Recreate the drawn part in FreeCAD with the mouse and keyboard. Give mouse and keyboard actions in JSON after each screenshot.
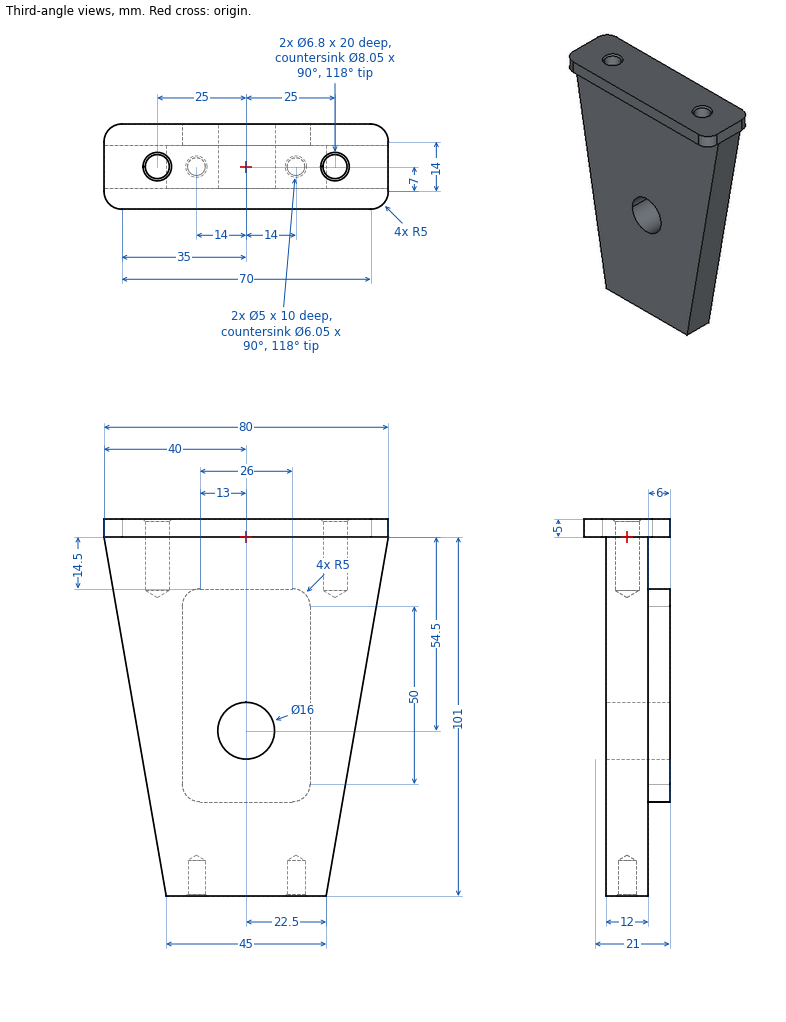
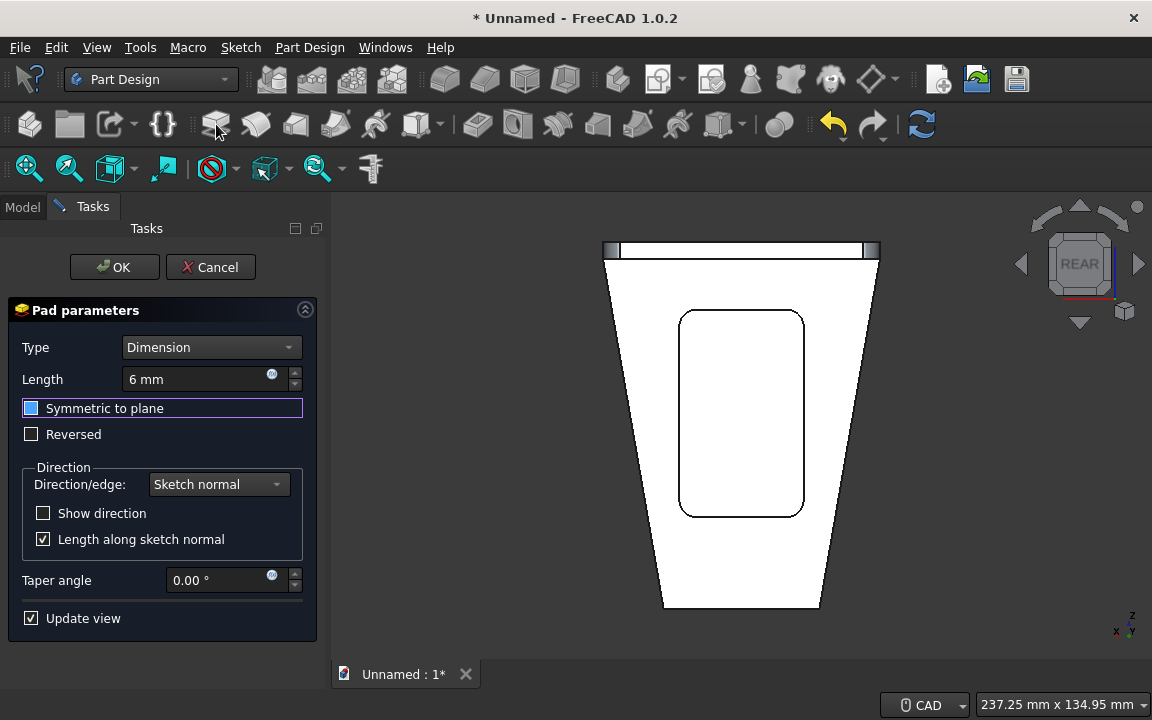
{"action": "left_click", "coordinate": [115, 267]}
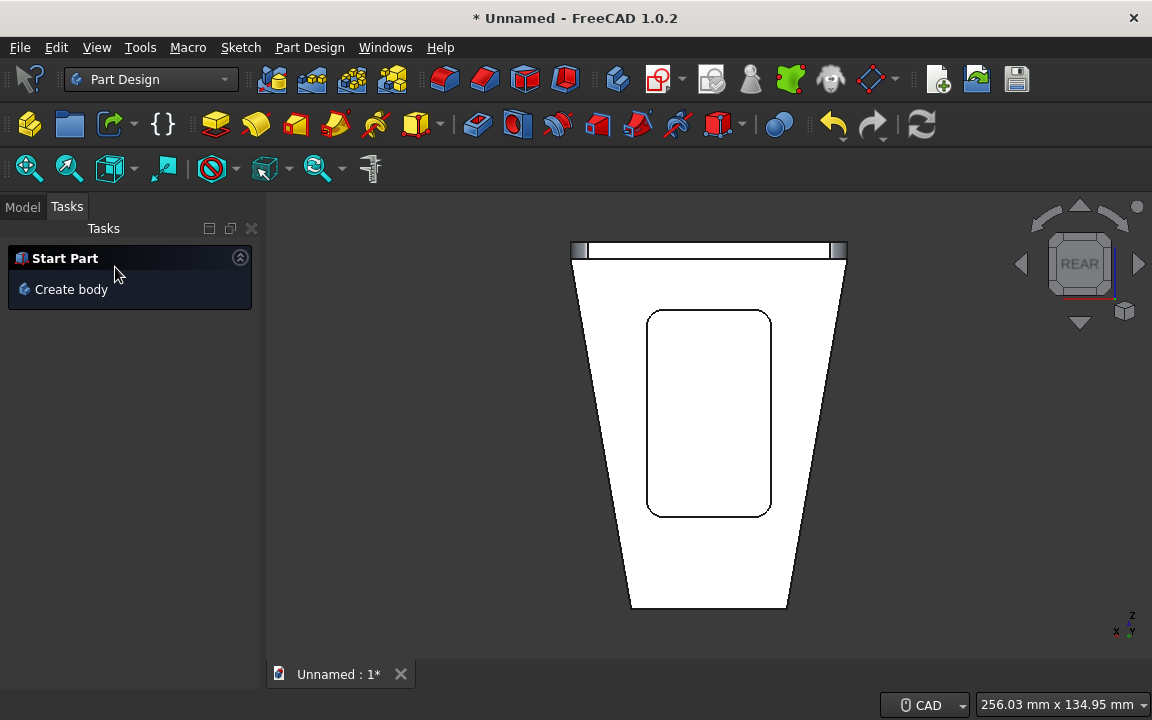
{"action": "left_click", "coordinate": [709, 383]}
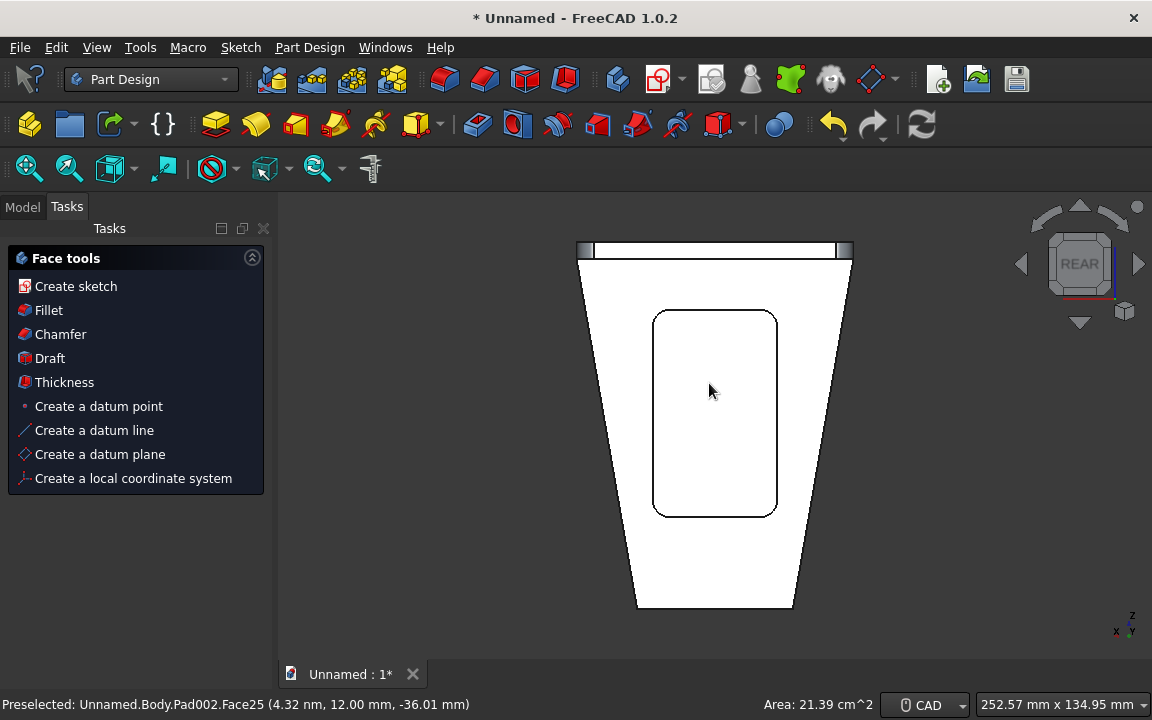
{"action": "left_click", "coordinate": [658, 80]}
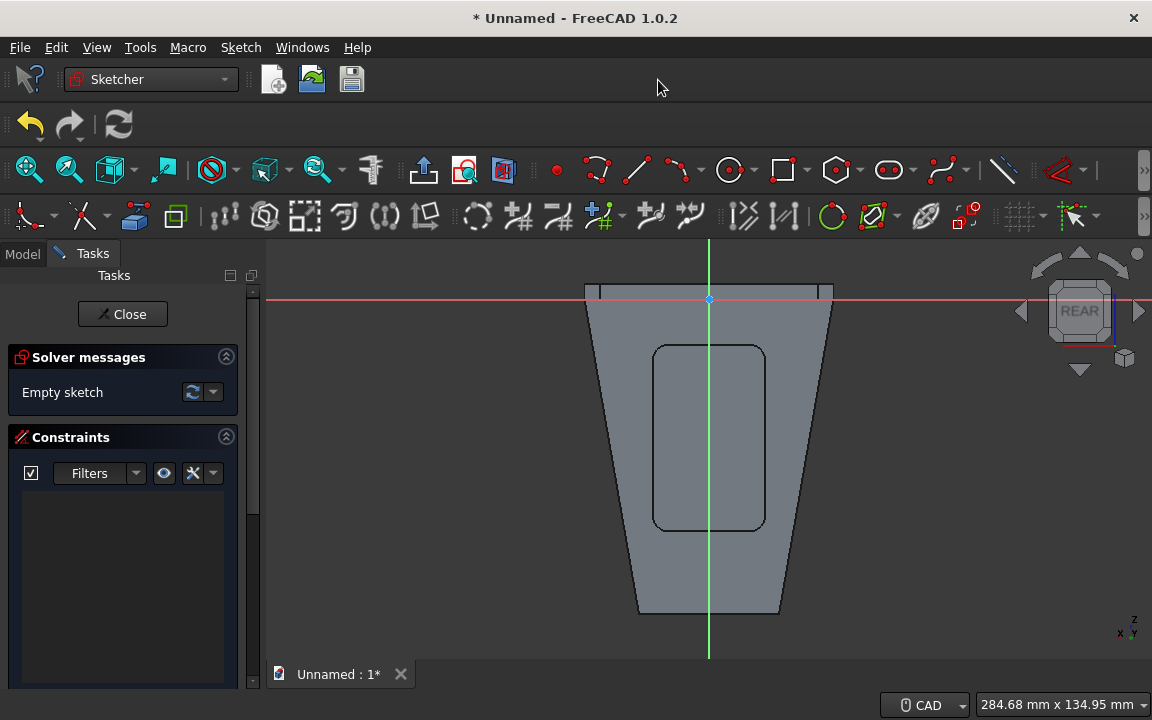
{"action": "scroll", "coordinate": [726, 474], "scroll_direction": "up", "scroll_amount": 8}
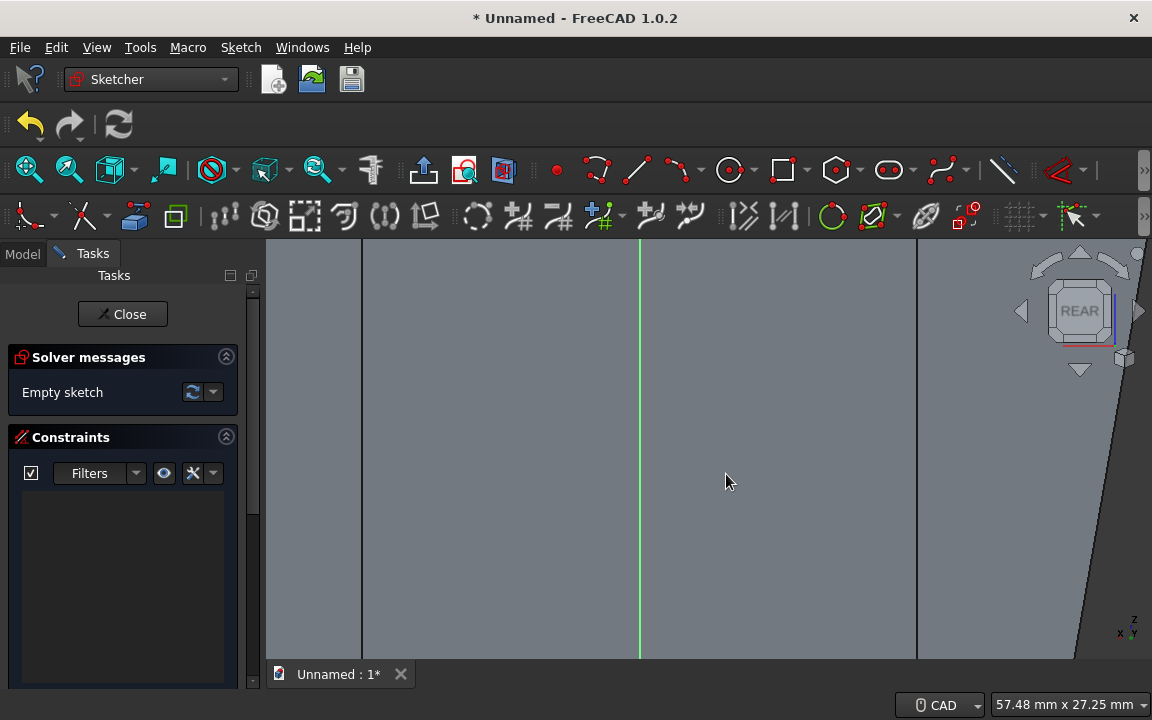
{"action": "left_click", "coordinate": [730, 170]}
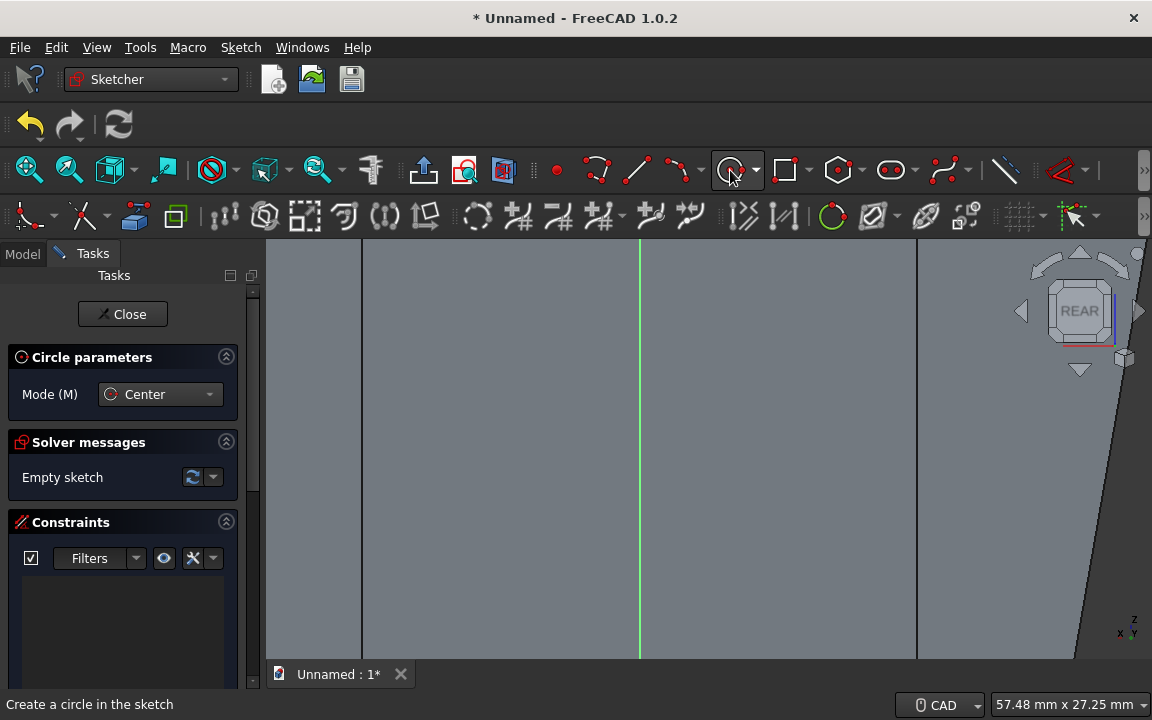
{"action": "left_click", "coordinate": [640, 448]}
{"action": "mouse_move", "coordinate": [727, 361]}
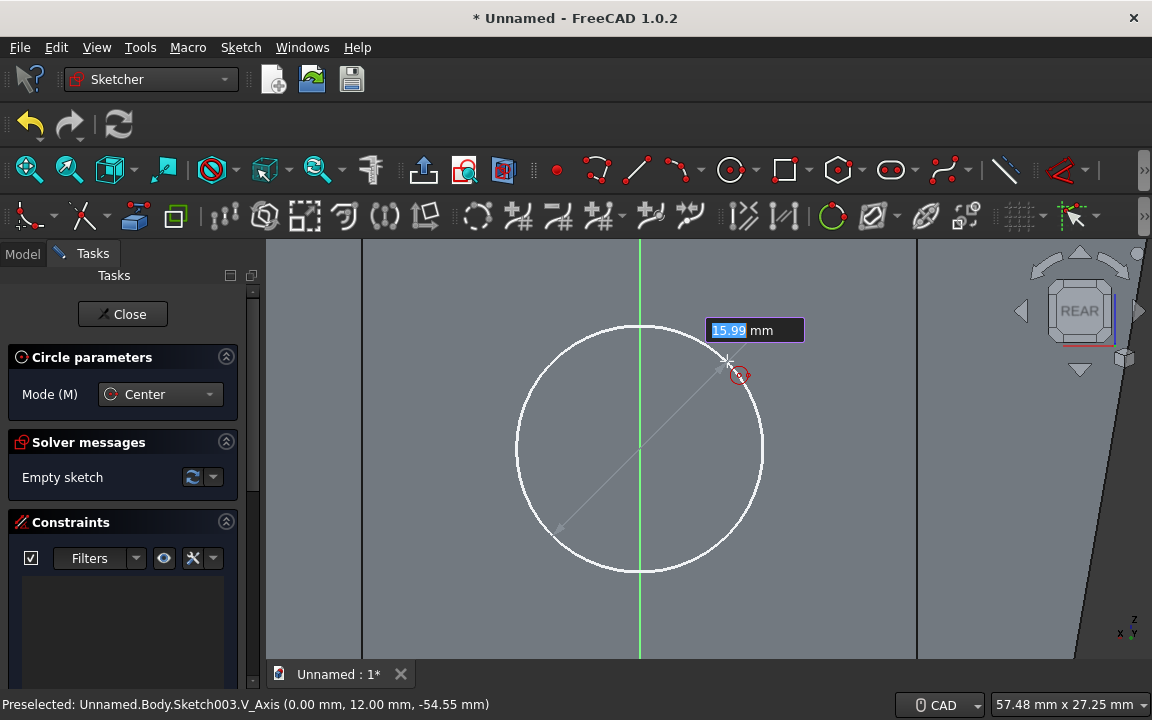
{"action": "type", "text": "16"}
{"action": "key", "text": "Return"}
{"action": "key", "text": "Escape"}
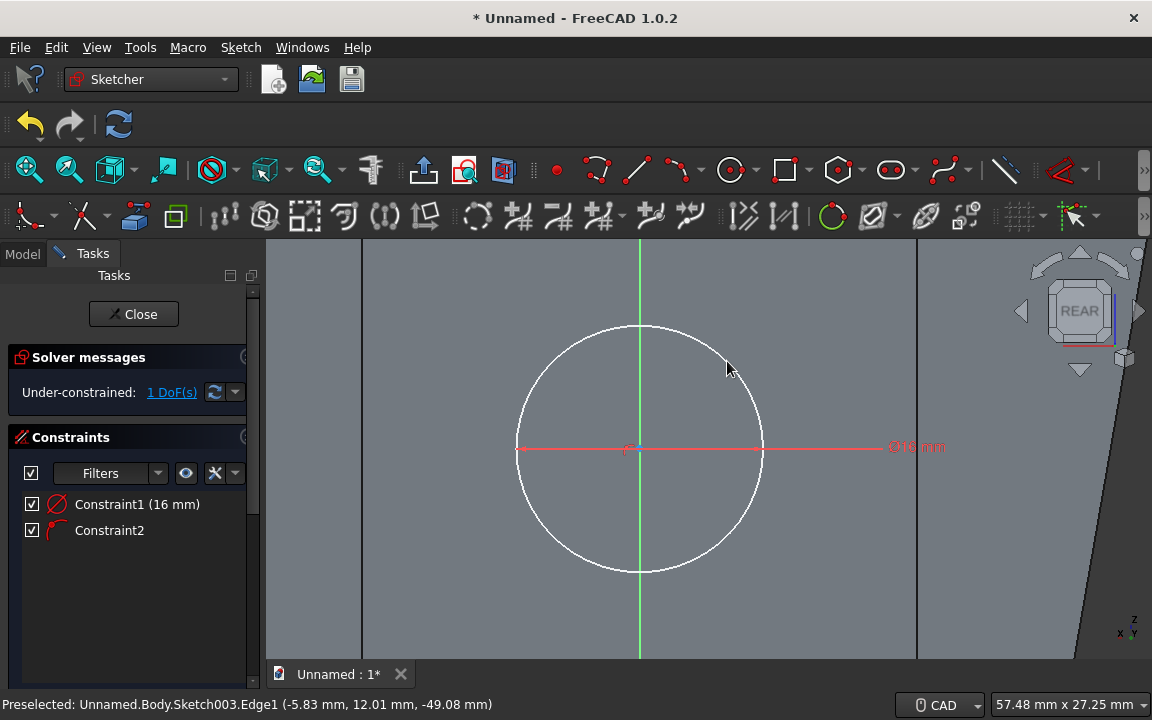
{"action": "left_click", "coordinate": [1060, 170]}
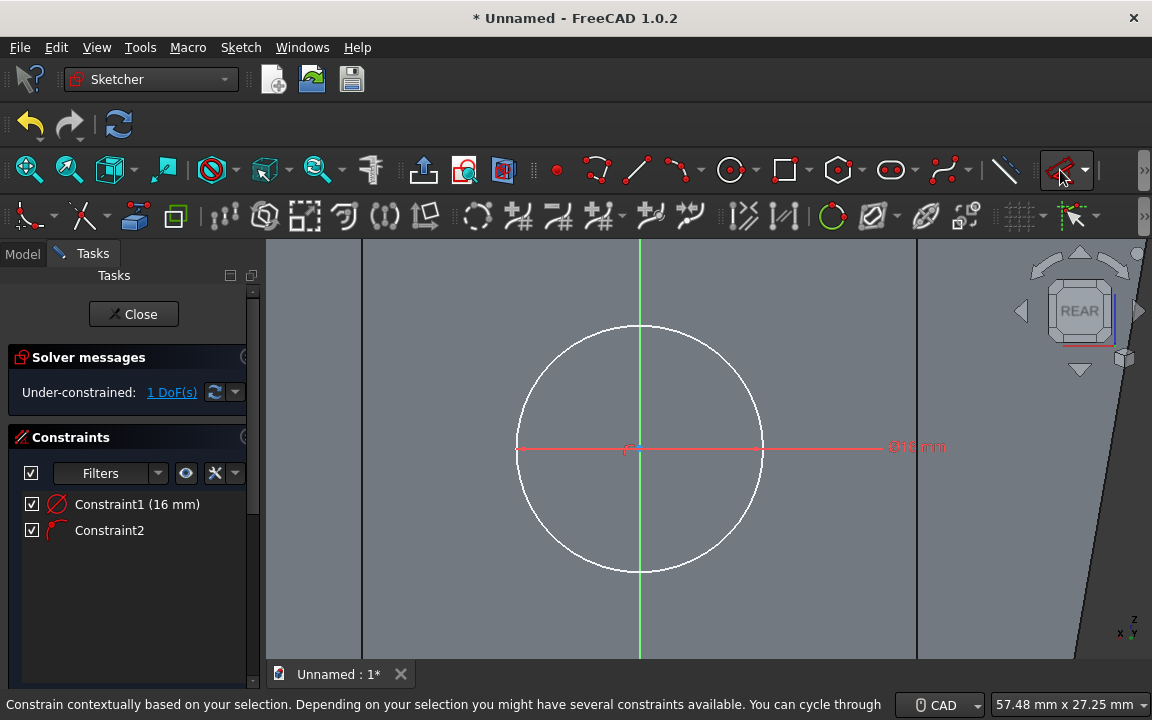
{"action": "left_click", "coordinate": [640, 449]}
{"action": "left_click", "coordinate": [674, 358]}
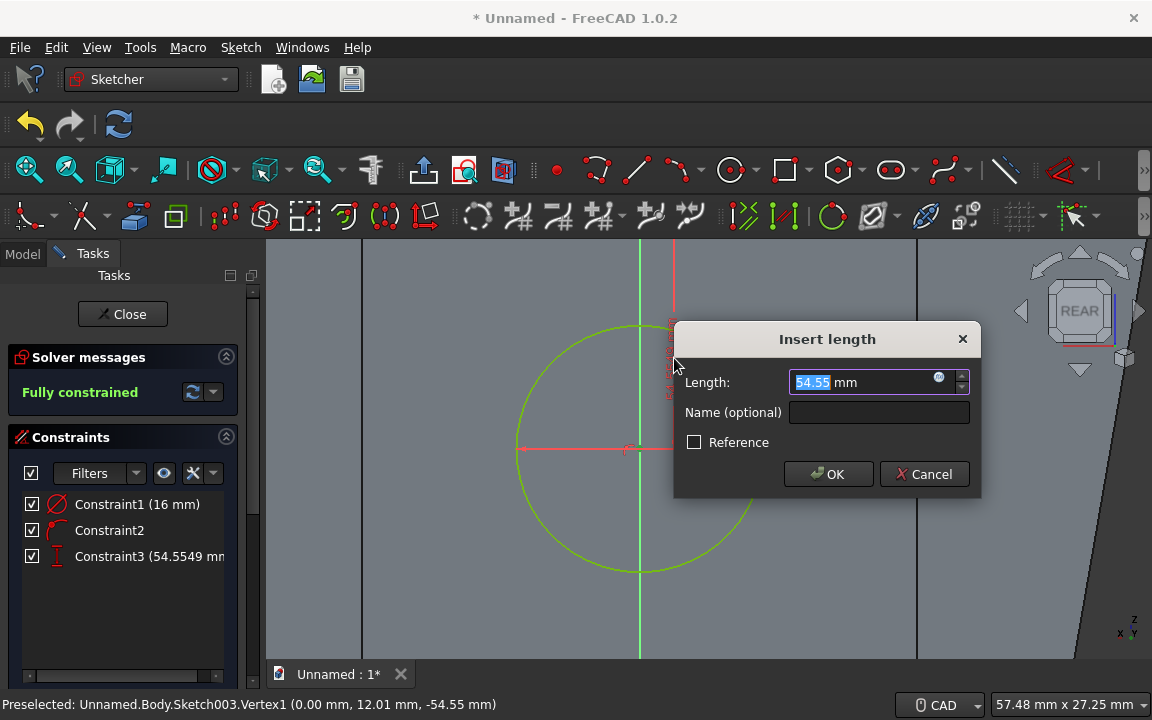
{"action": "type", "text": "54.5"}
{"action": "key", "text": "Return"}
{"action": "key", "text": "Escape"}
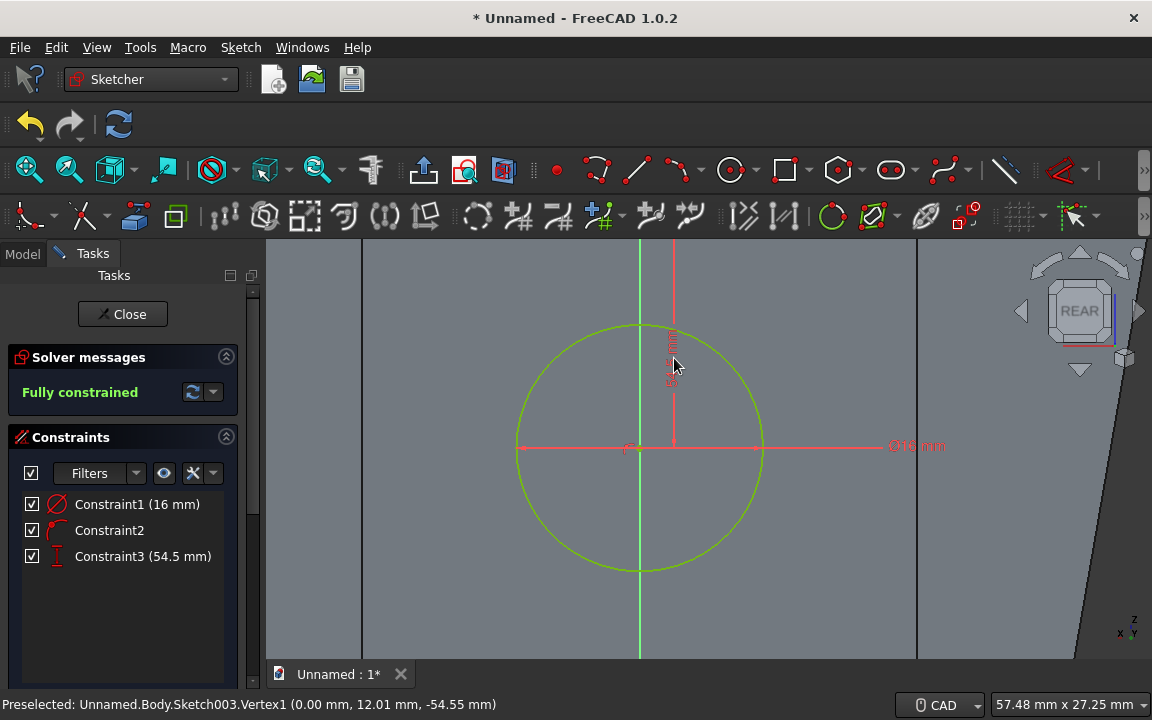
{"action": "left_click", "coordinate": [123, 314]}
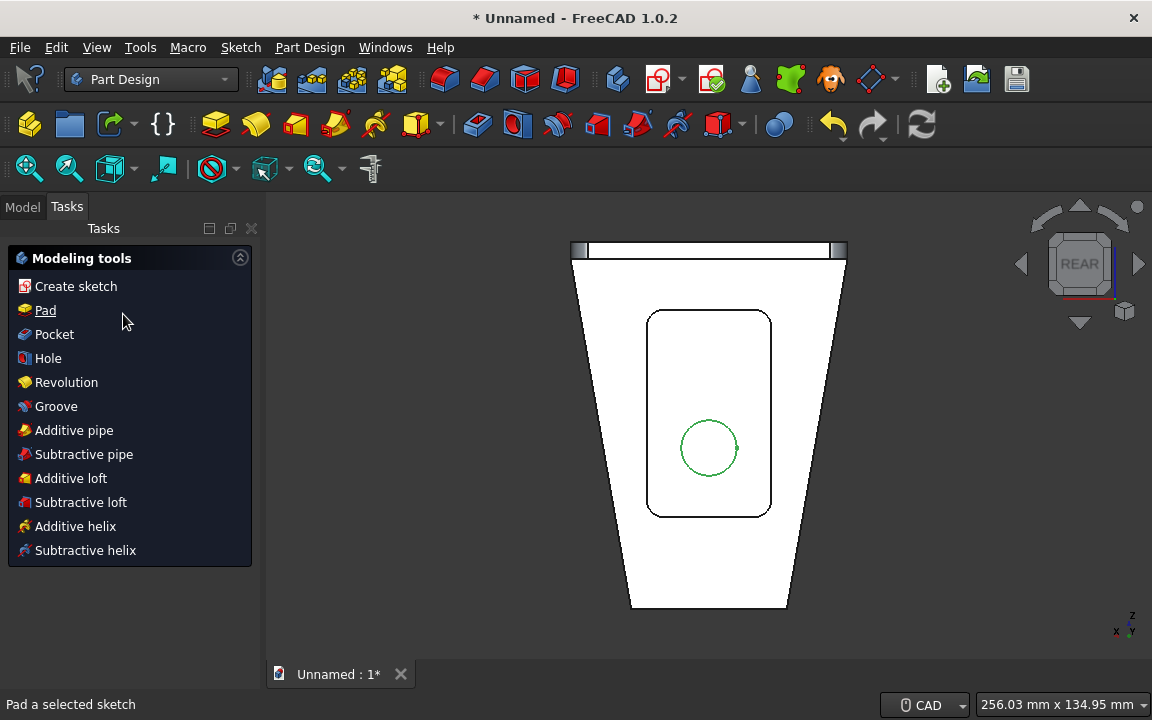
{"action": "left_click", "coordinate": [478, 124]}